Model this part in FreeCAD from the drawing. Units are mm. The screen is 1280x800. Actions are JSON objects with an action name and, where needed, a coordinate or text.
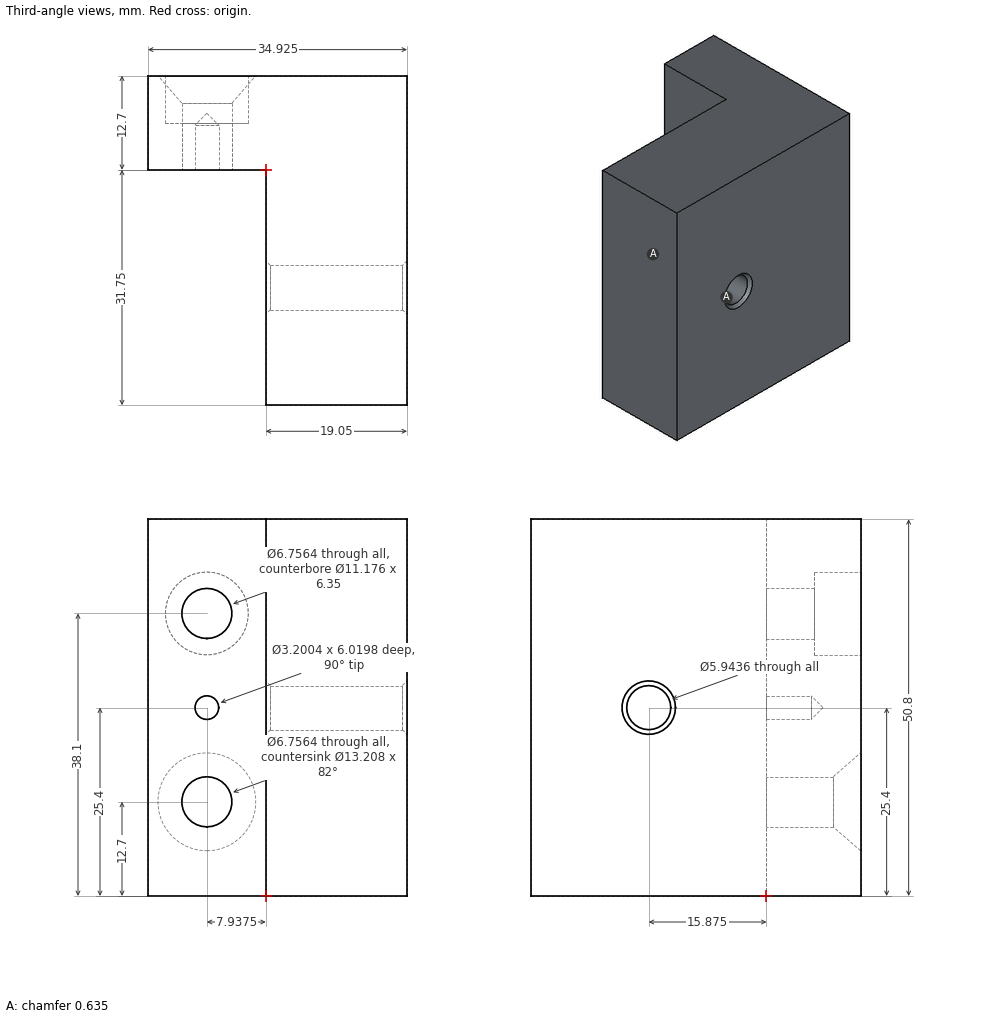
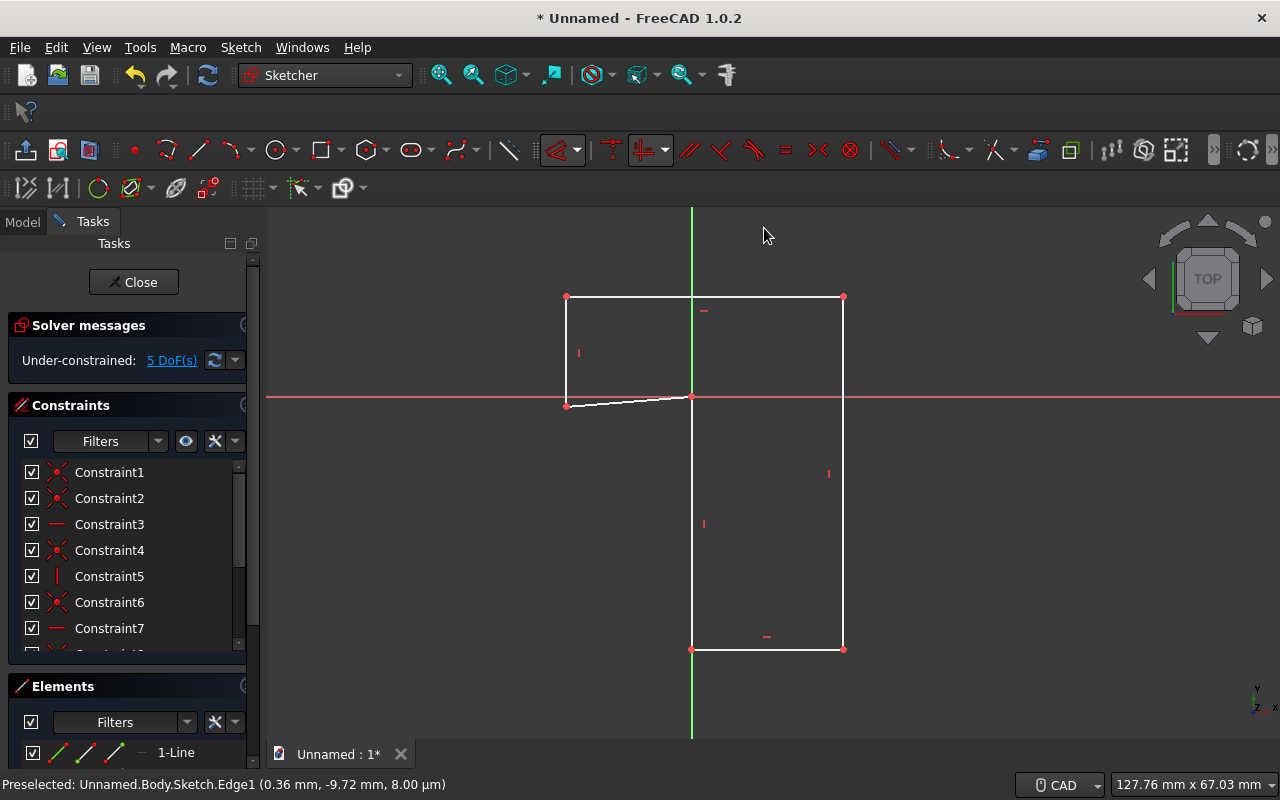
{"action": "left_click", "coordinate": [654, 400]}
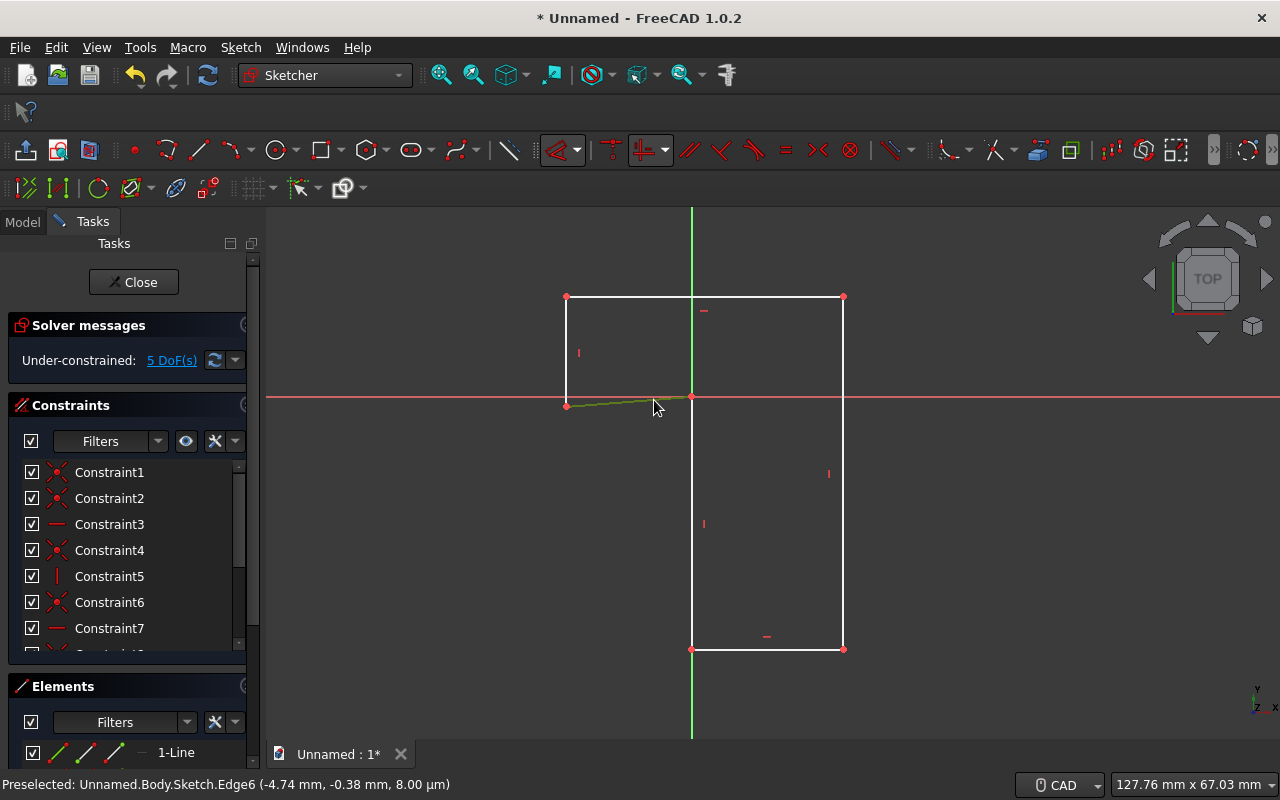
{"action": "left_click", "coordinate": [668, 150]}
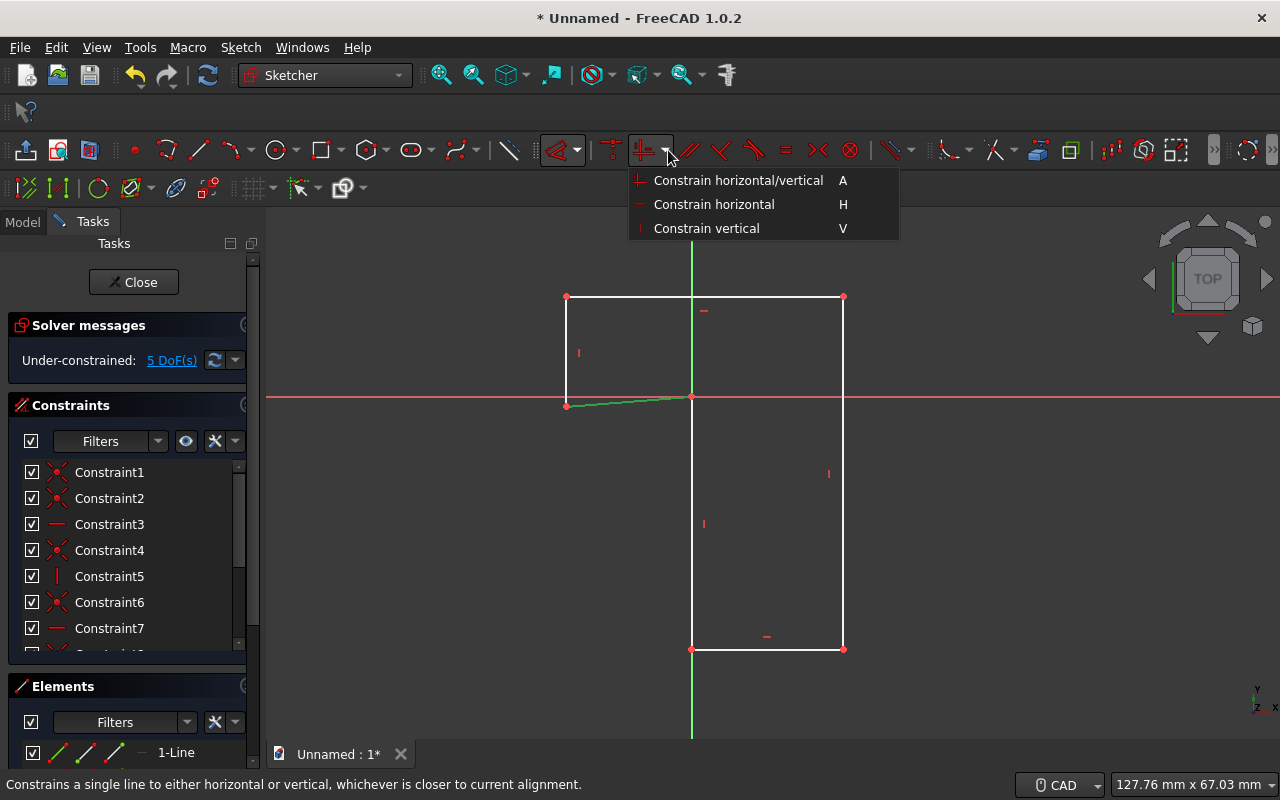
{"action": "left_click", "coordinate": [764, 204]}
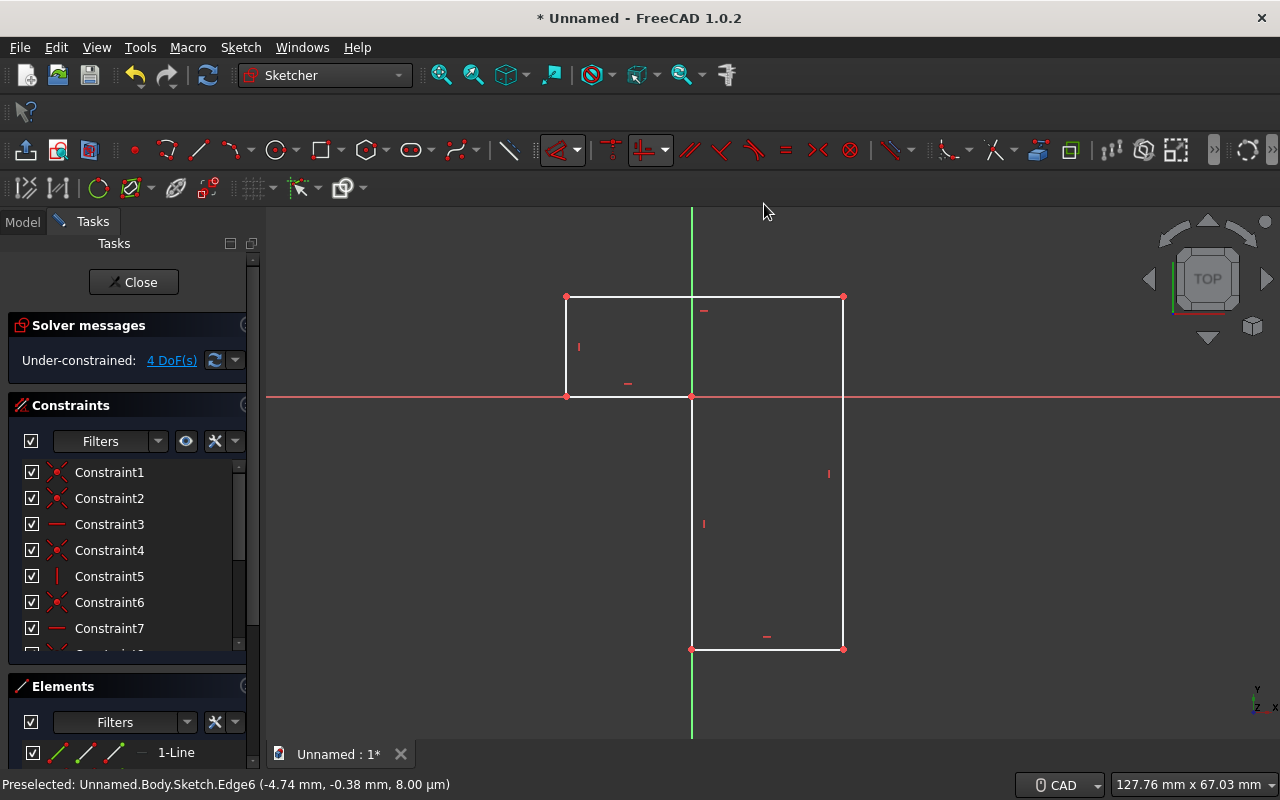
{"action": "left_click", "coordinate": [566, 327]}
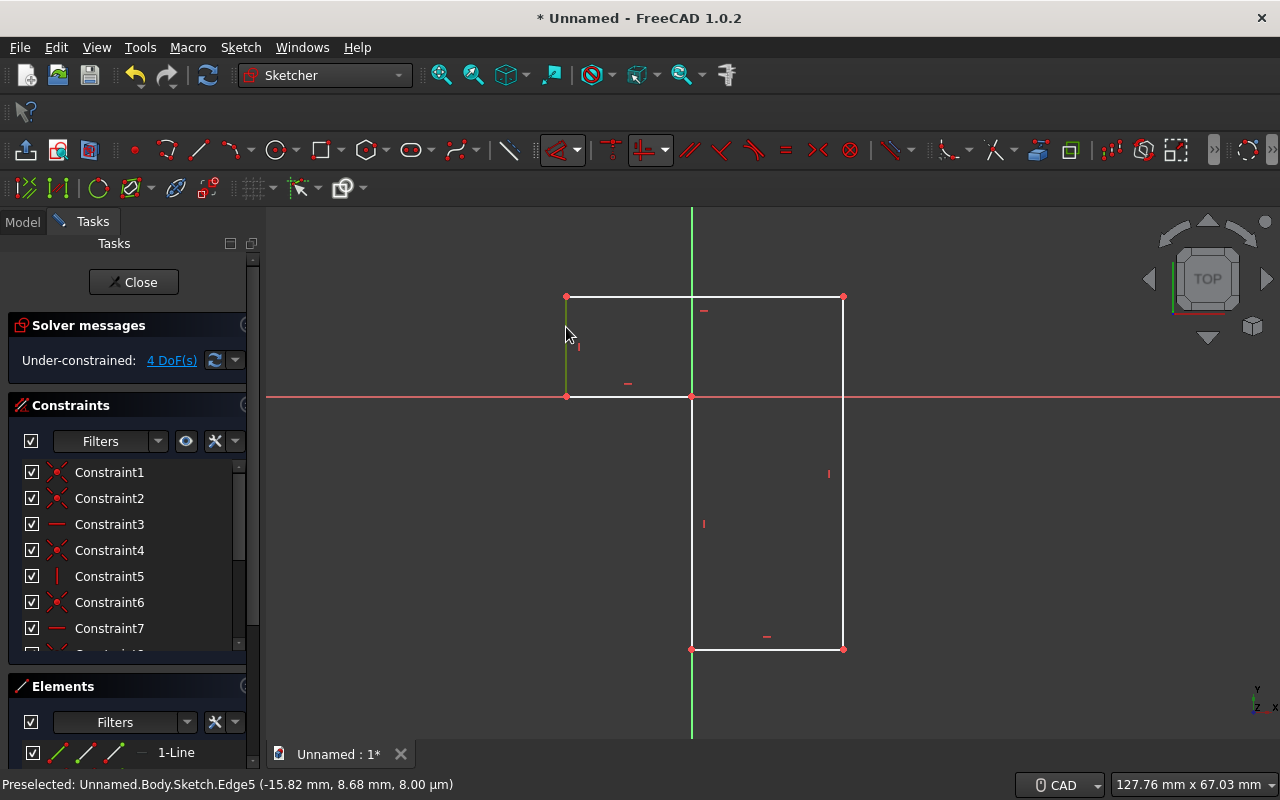
{"action": "left_click", "coordinate": [580, 150]}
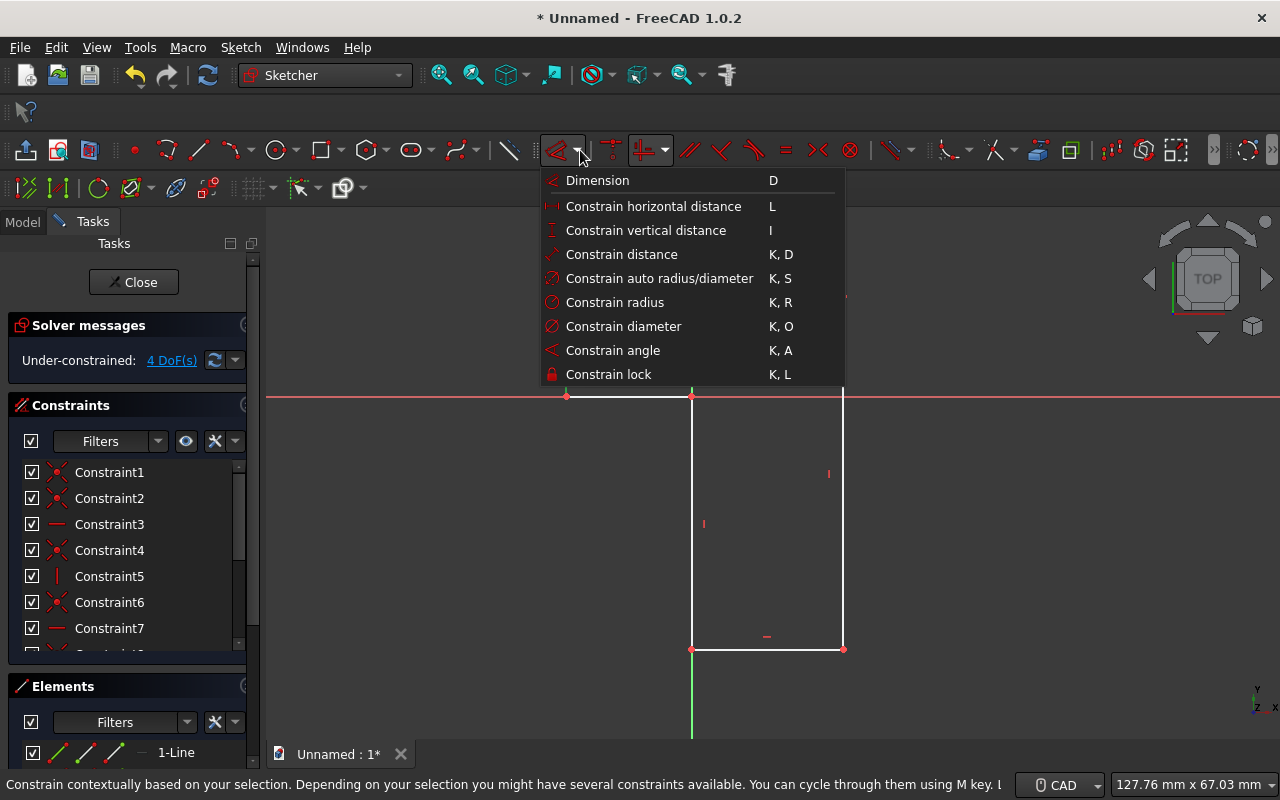
{"action": "left_click", "coordinate": [693, 230]}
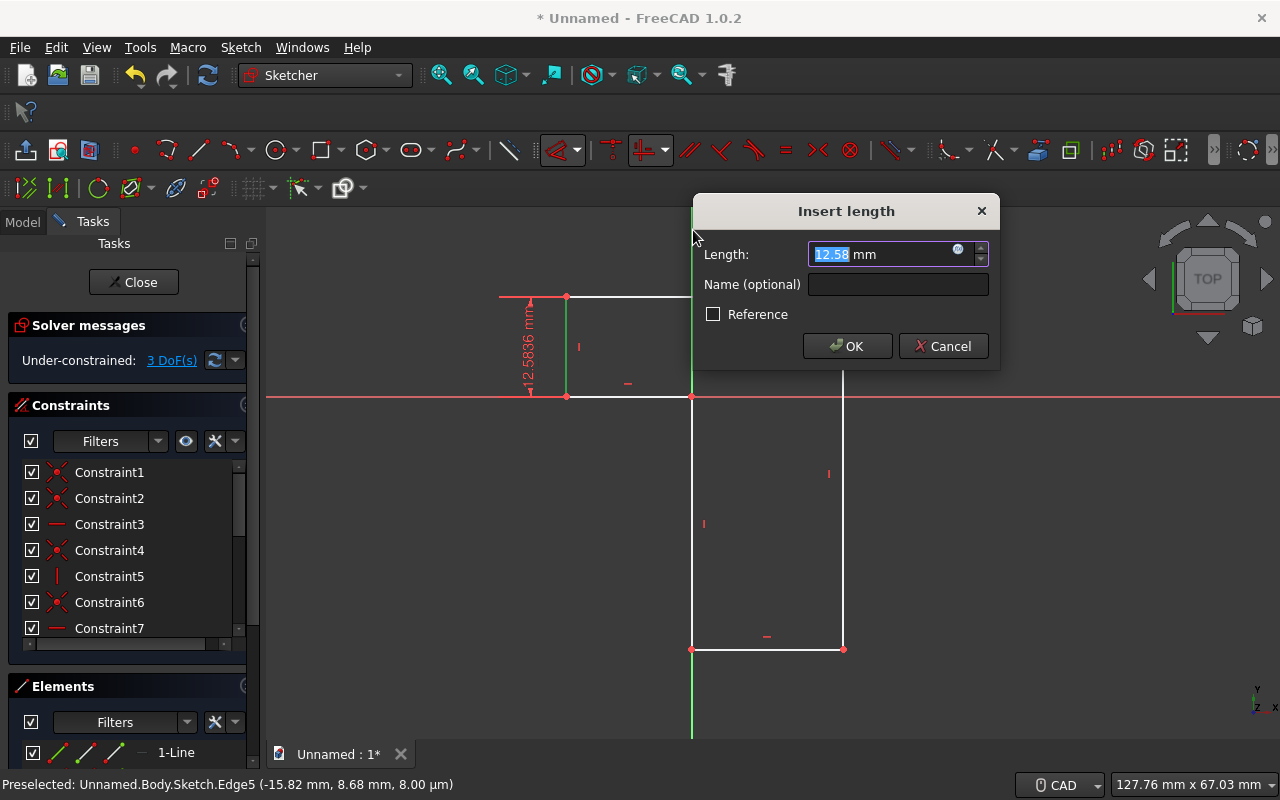
{"action": "type", "text": "12.7"}
{"action": "key", "text": "Return"}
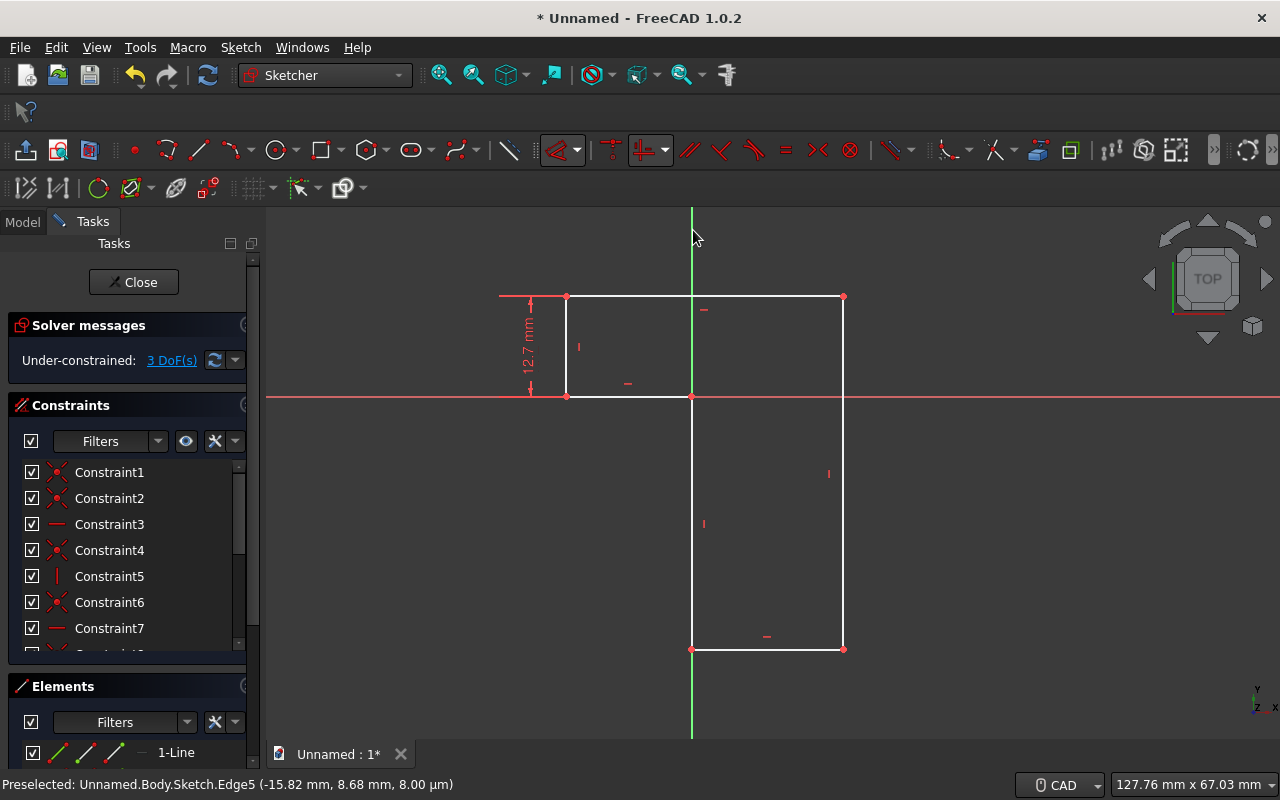
{"action": "left_click", "coordinate": [692, 473]}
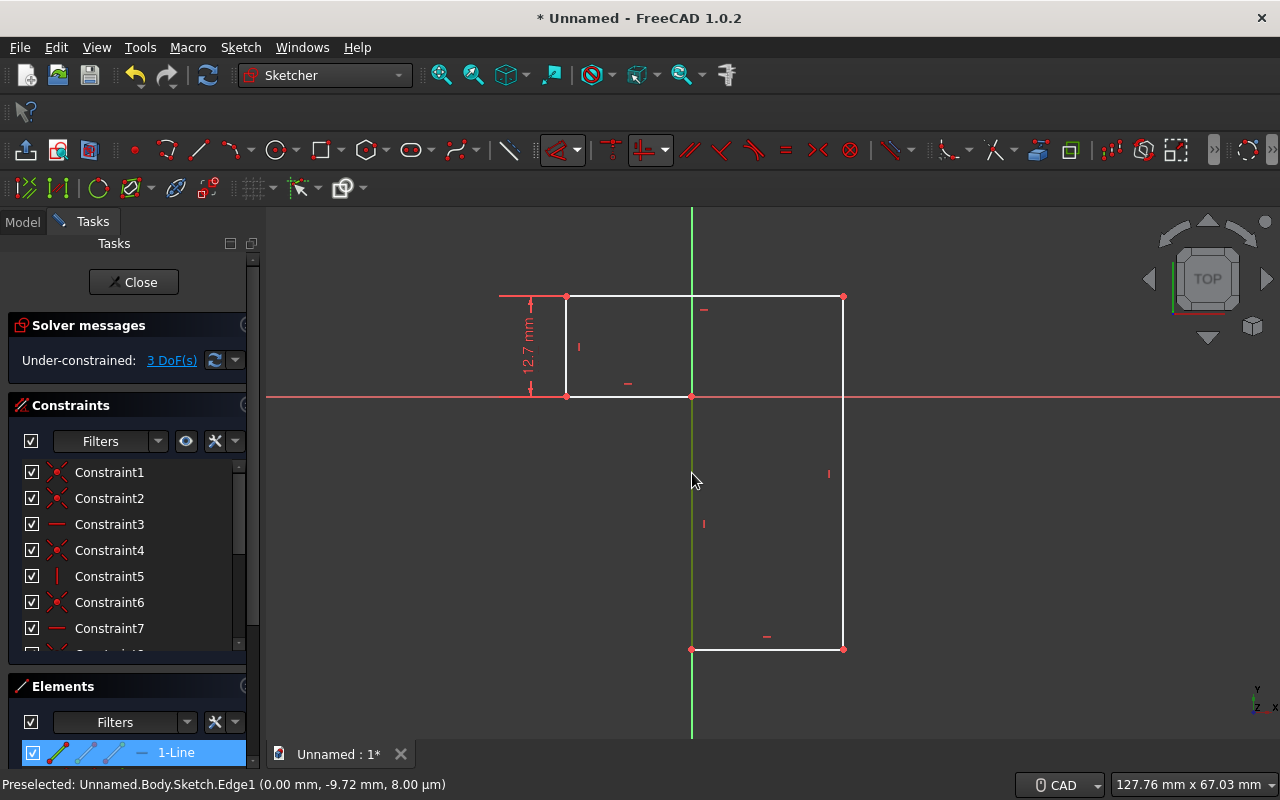
{"action": "left_click", "coordinate": [580, 150]}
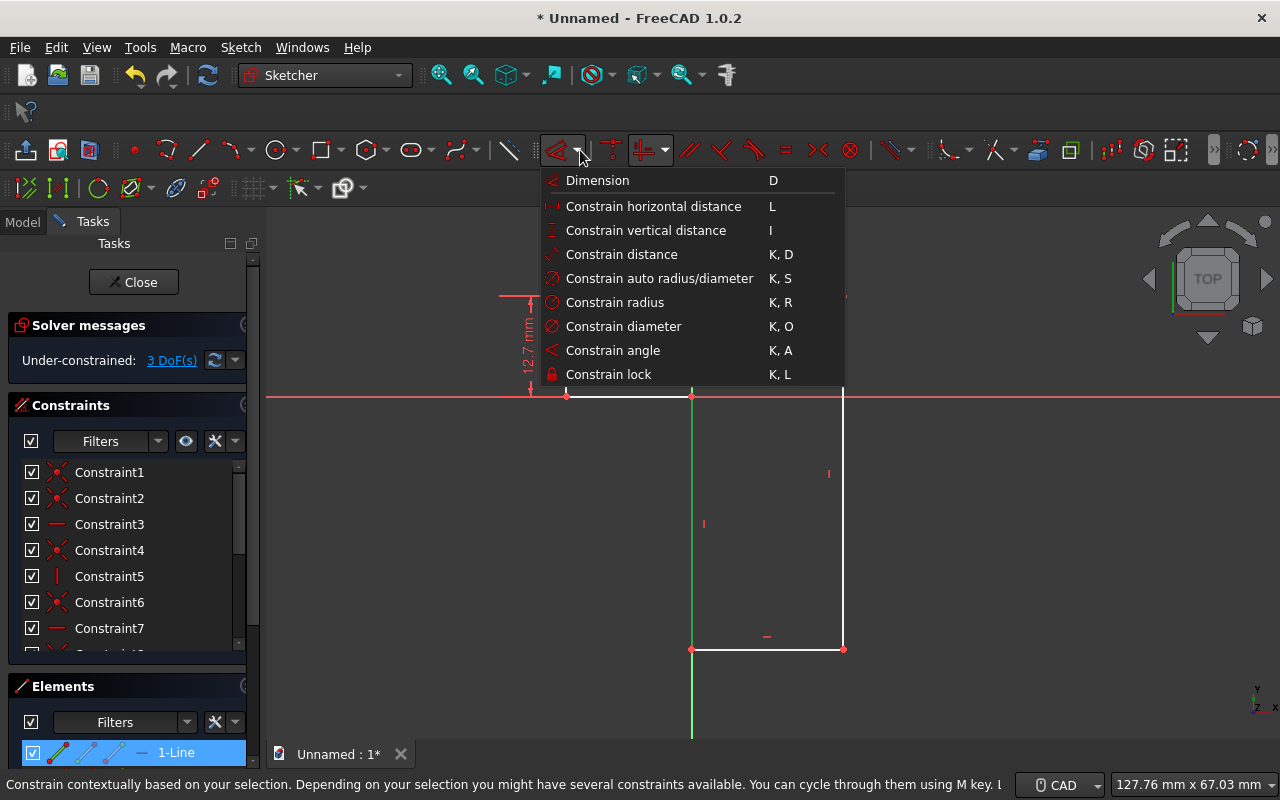
{"action": "left_click", "coordinate": [693, 230]}